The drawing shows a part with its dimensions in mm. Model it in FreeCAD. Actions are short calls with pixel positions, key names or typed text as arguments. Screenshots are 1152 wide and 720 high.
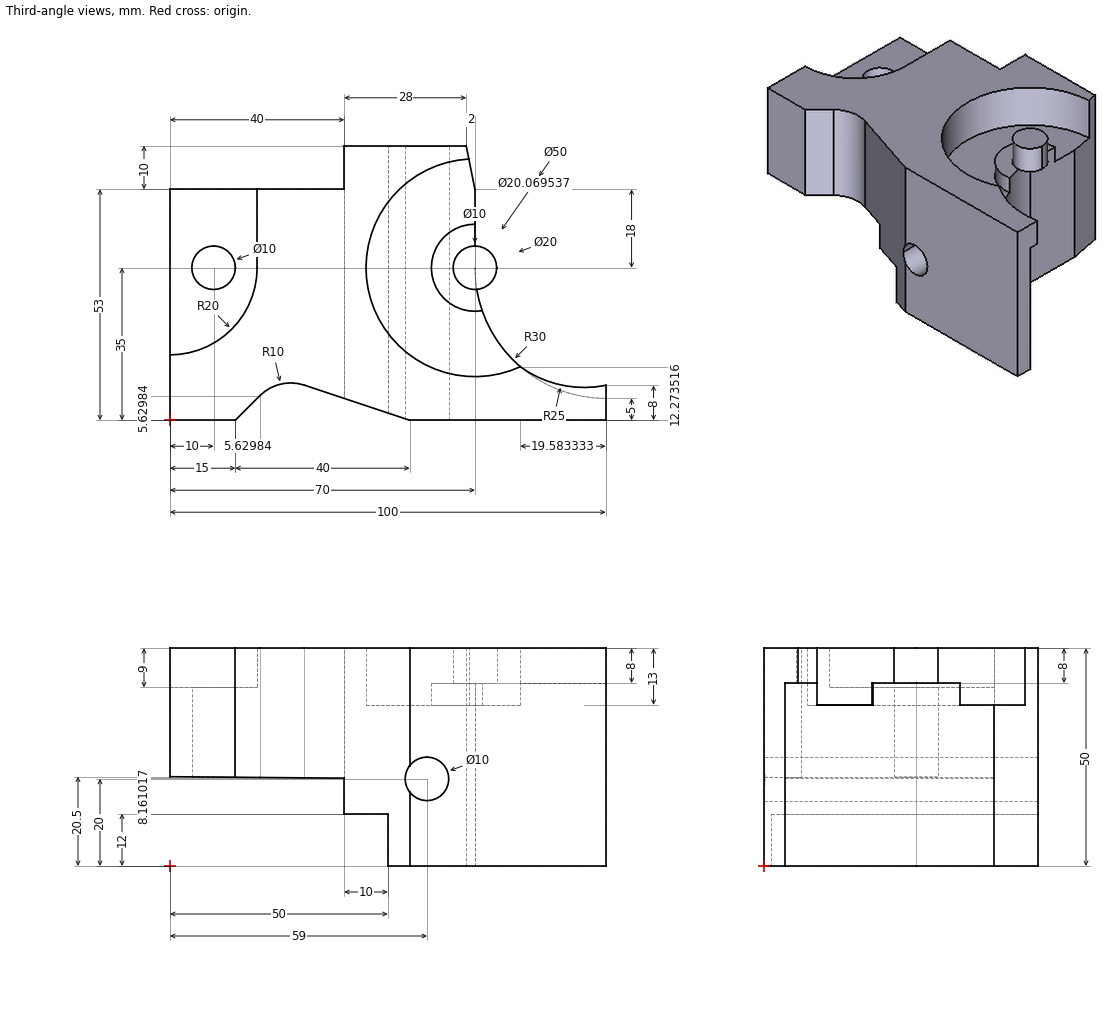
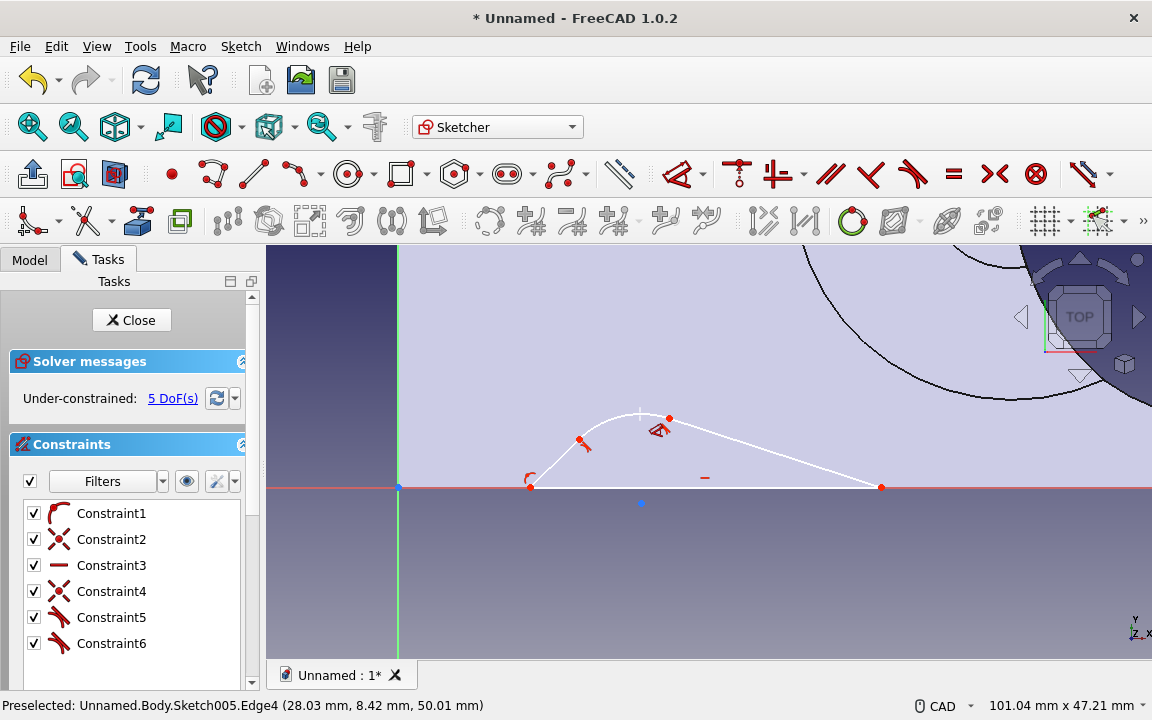
click(640, 414)
click(640, 382)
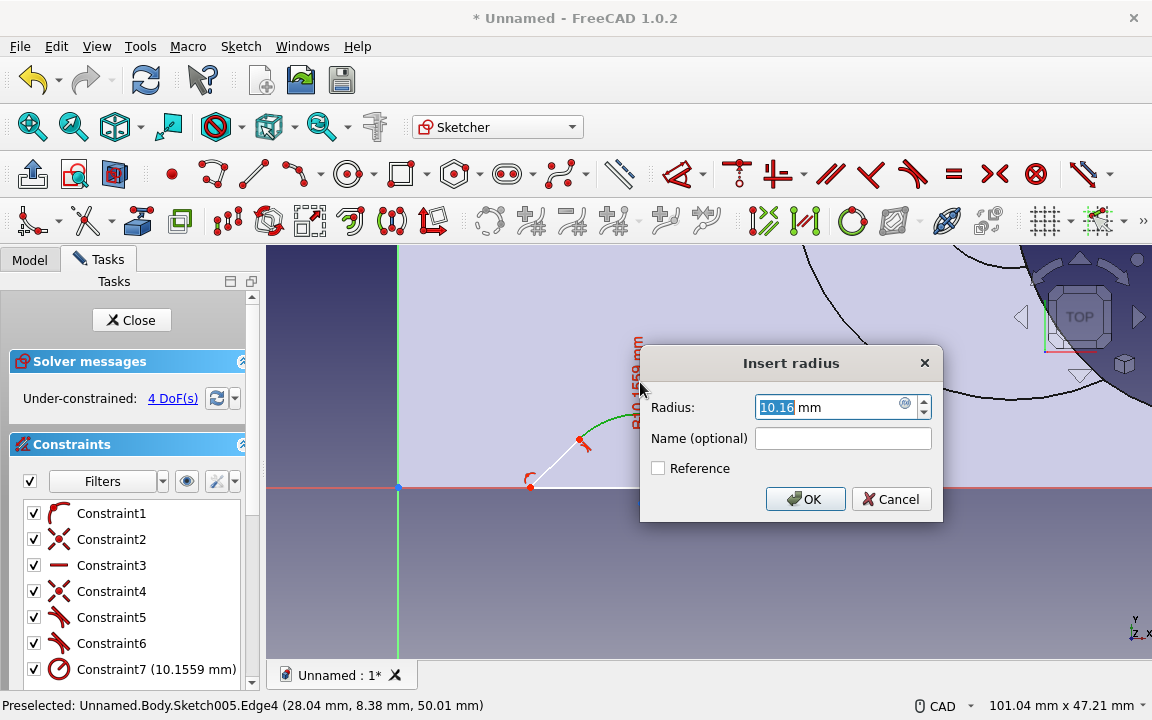
text(10)
key(Return)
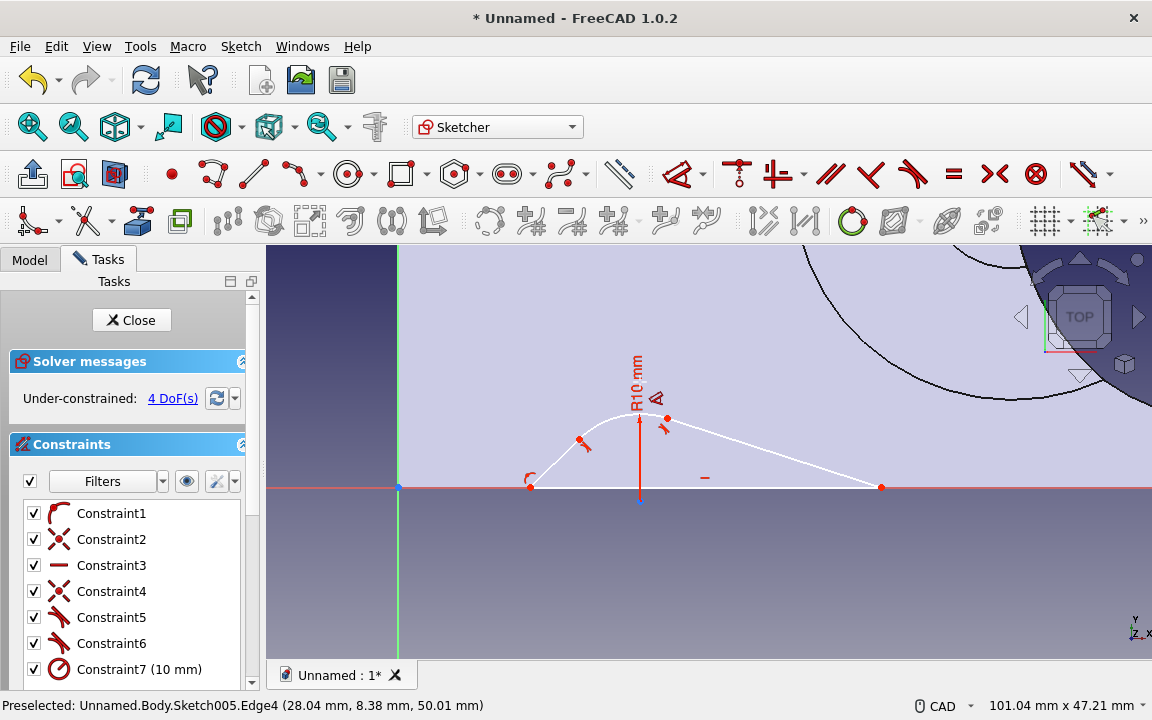
click(635, 488)
click(705, 522)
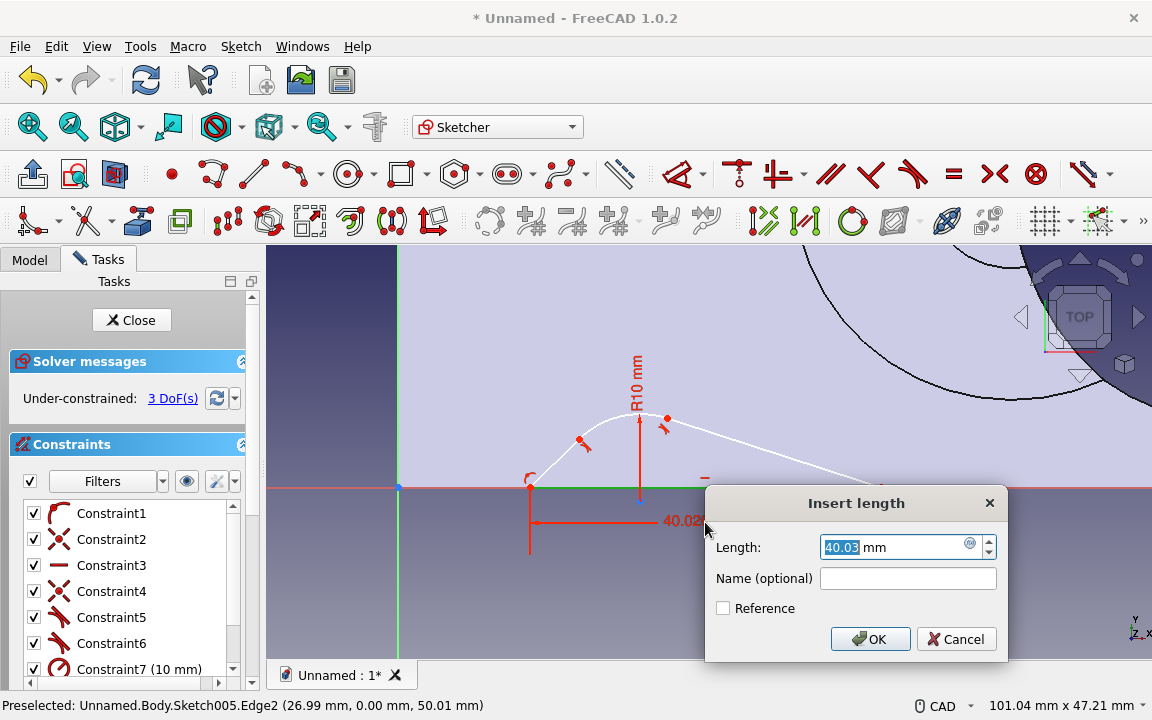
text(40)
key(Return)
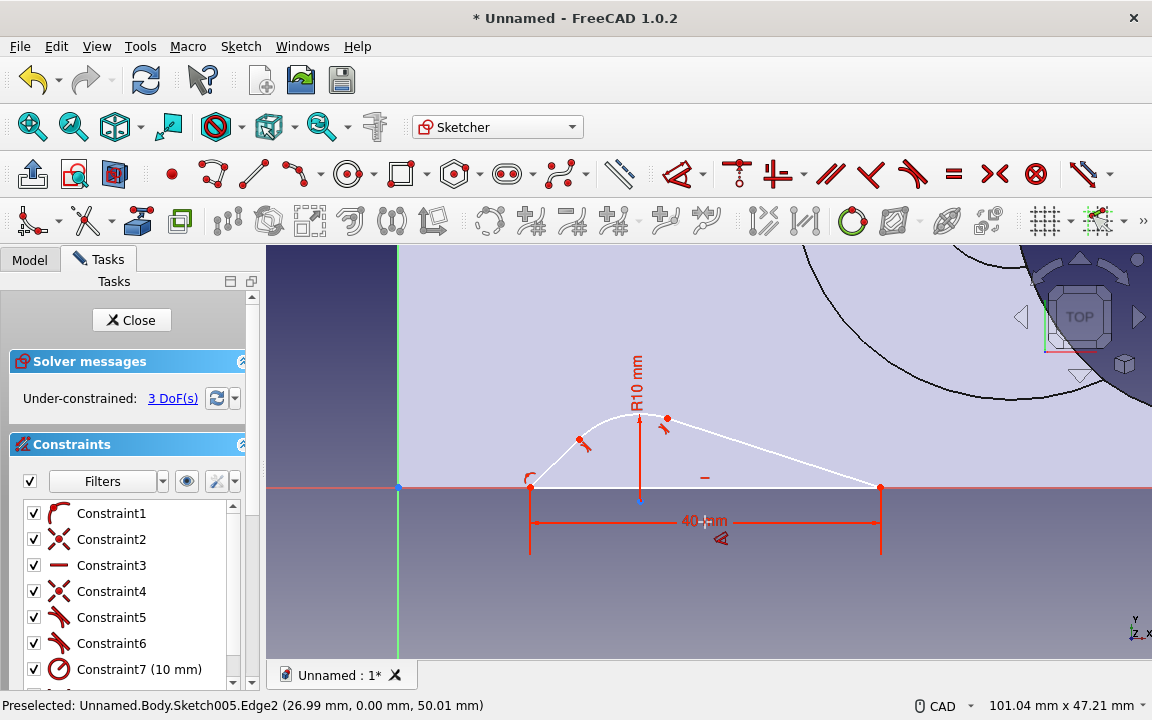
click(530, 488)
click(464, 522)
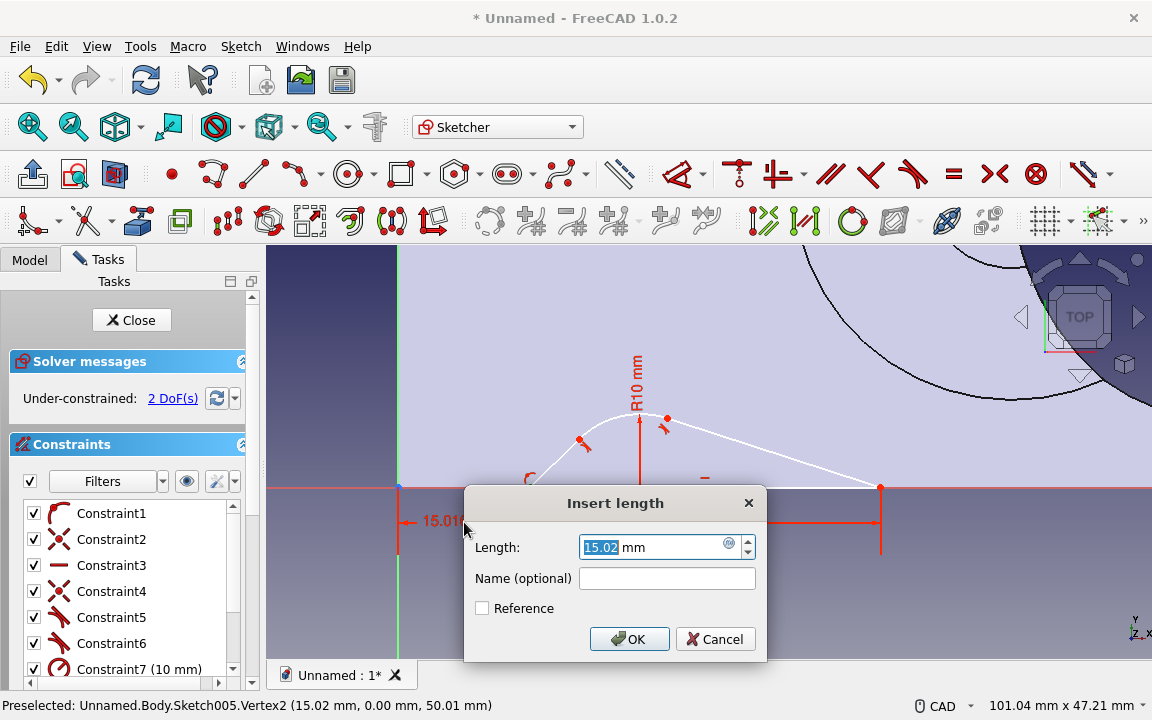
text(15)
key(Return)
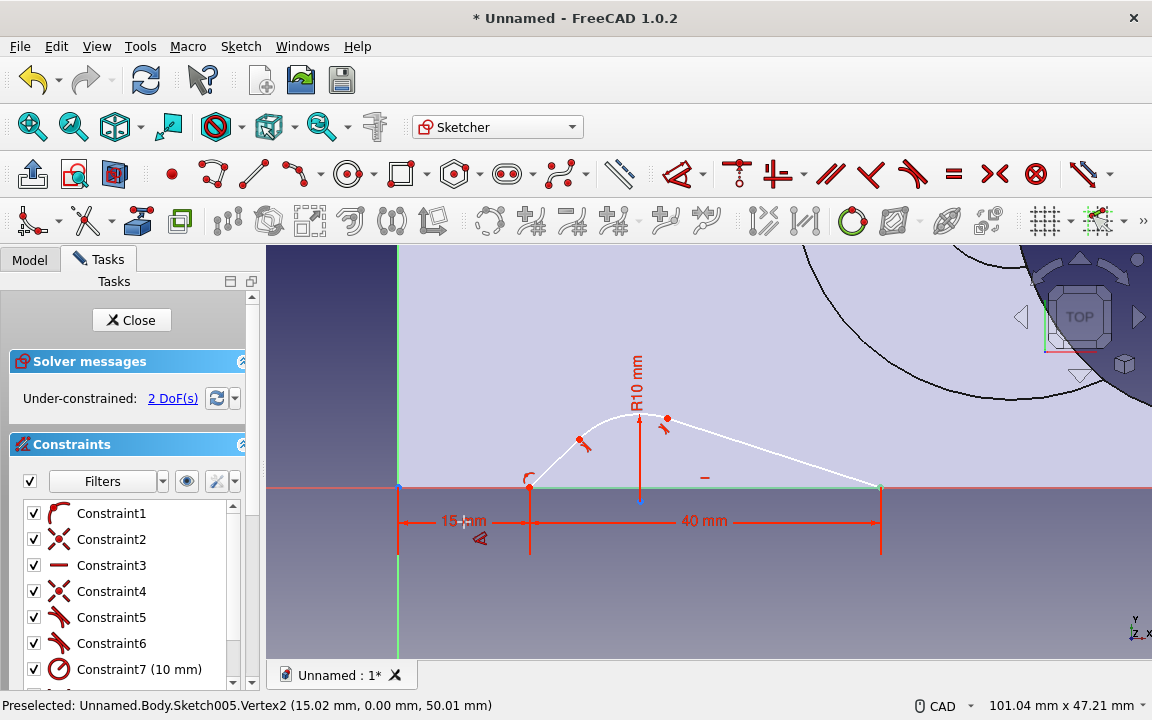
click(579, 439)
click(364, 463)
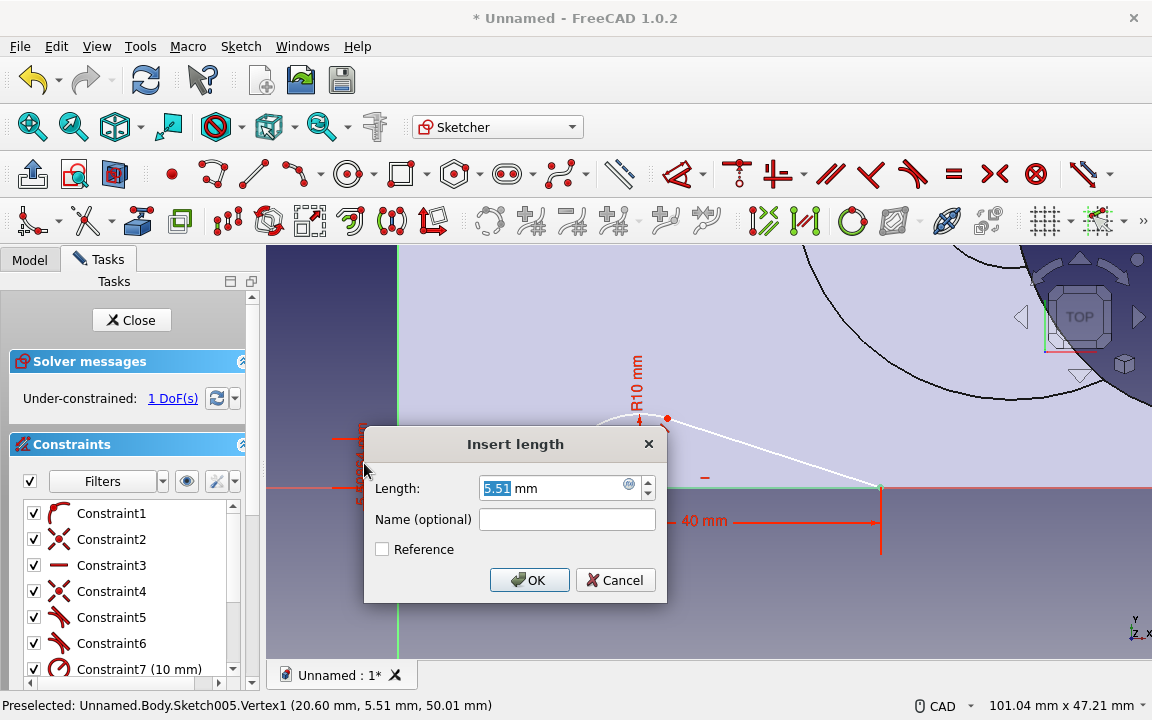
text(5.62984)
key(Return)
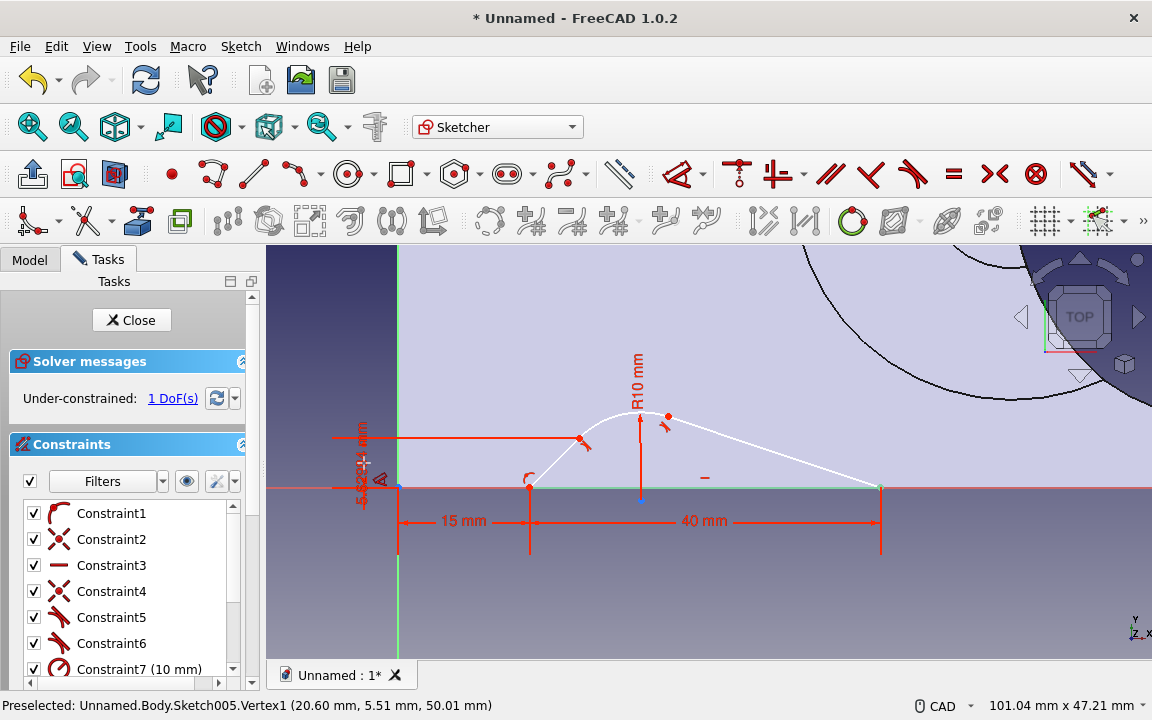
click(564, 453)
click(554, 522)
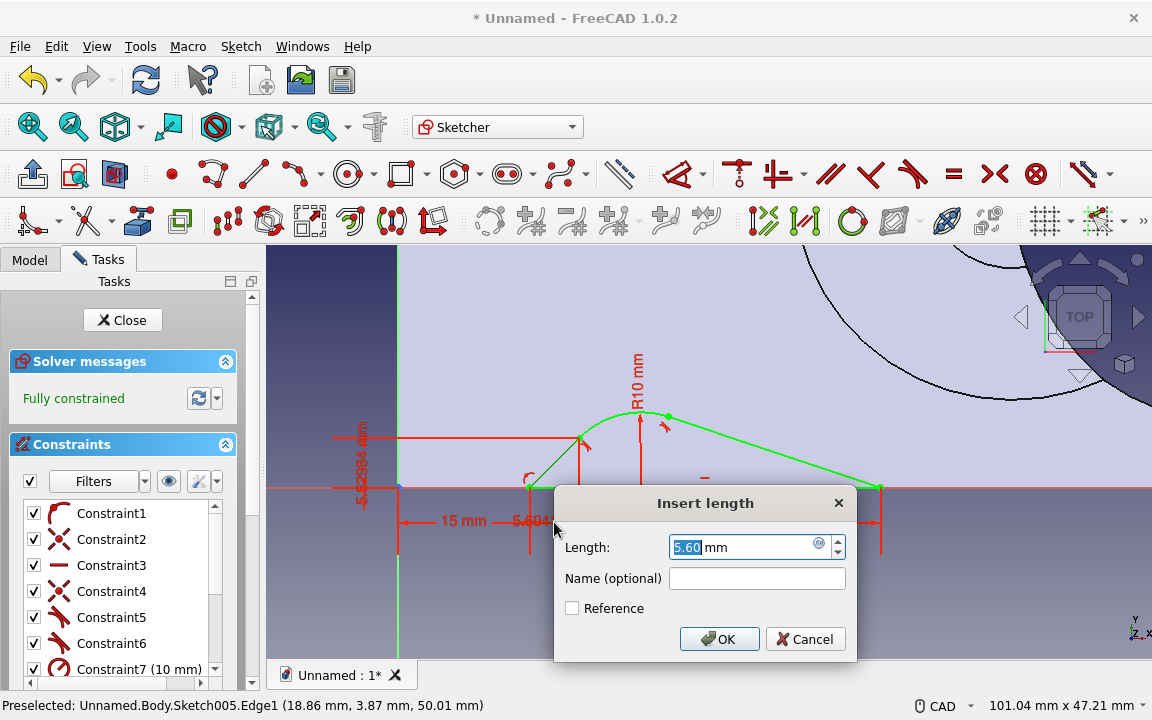
text(5.62984)
key(Return)
key(Escape)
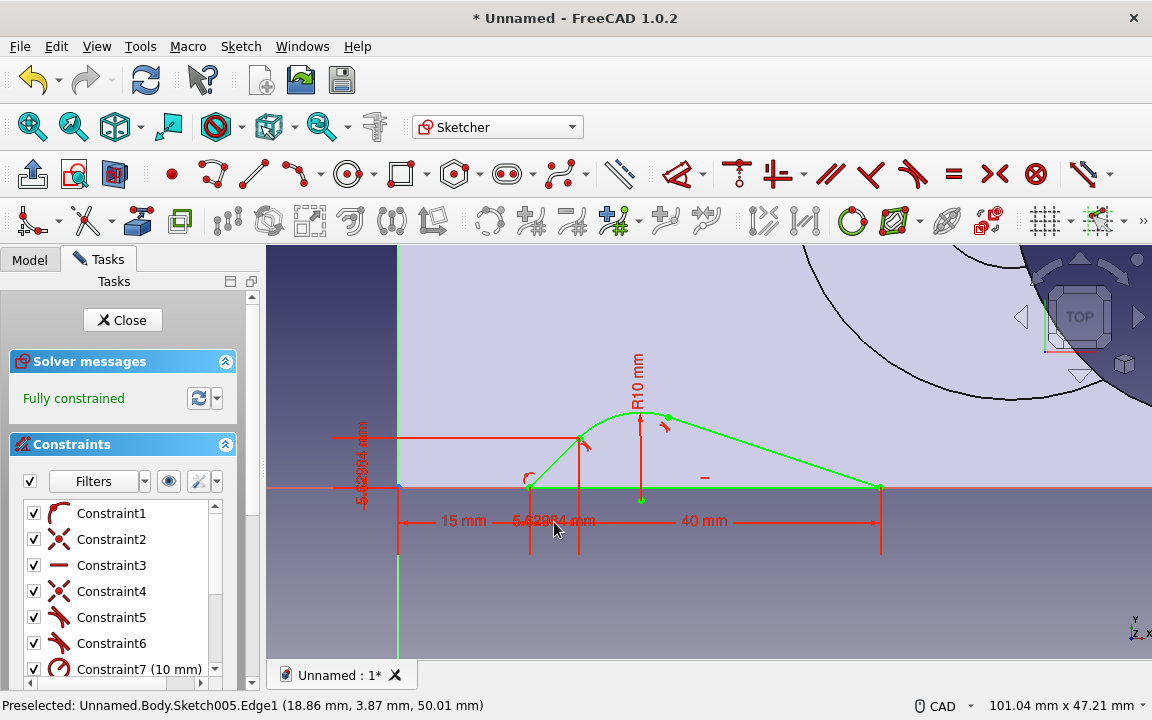
click(123, 320)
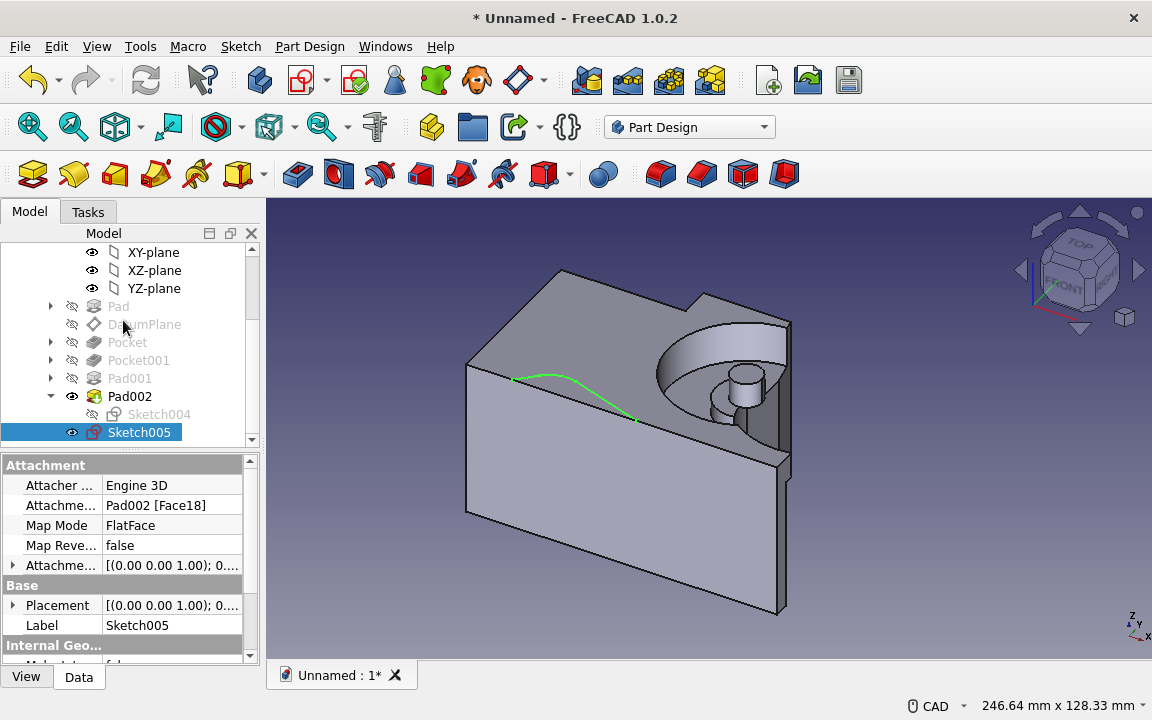
click(298, 174)